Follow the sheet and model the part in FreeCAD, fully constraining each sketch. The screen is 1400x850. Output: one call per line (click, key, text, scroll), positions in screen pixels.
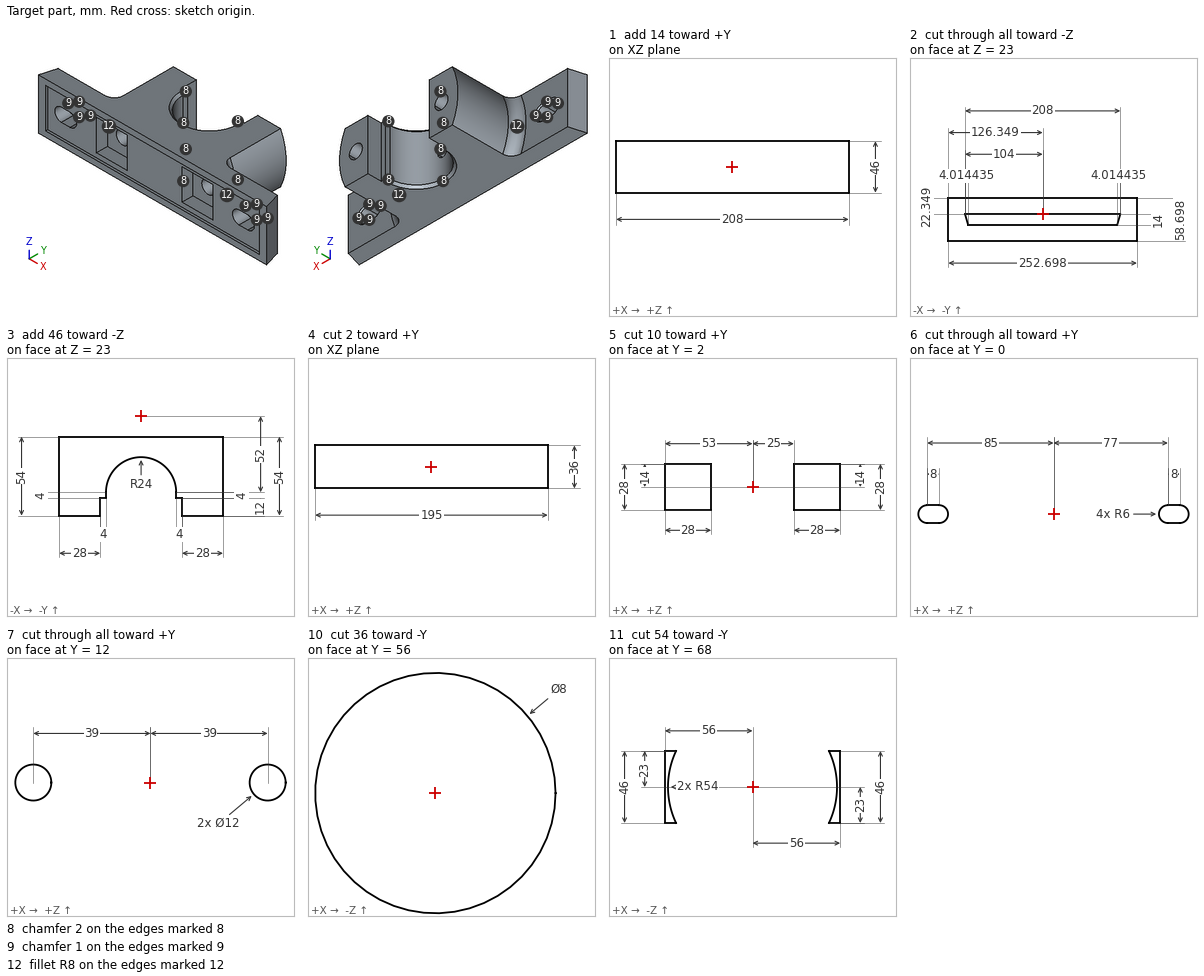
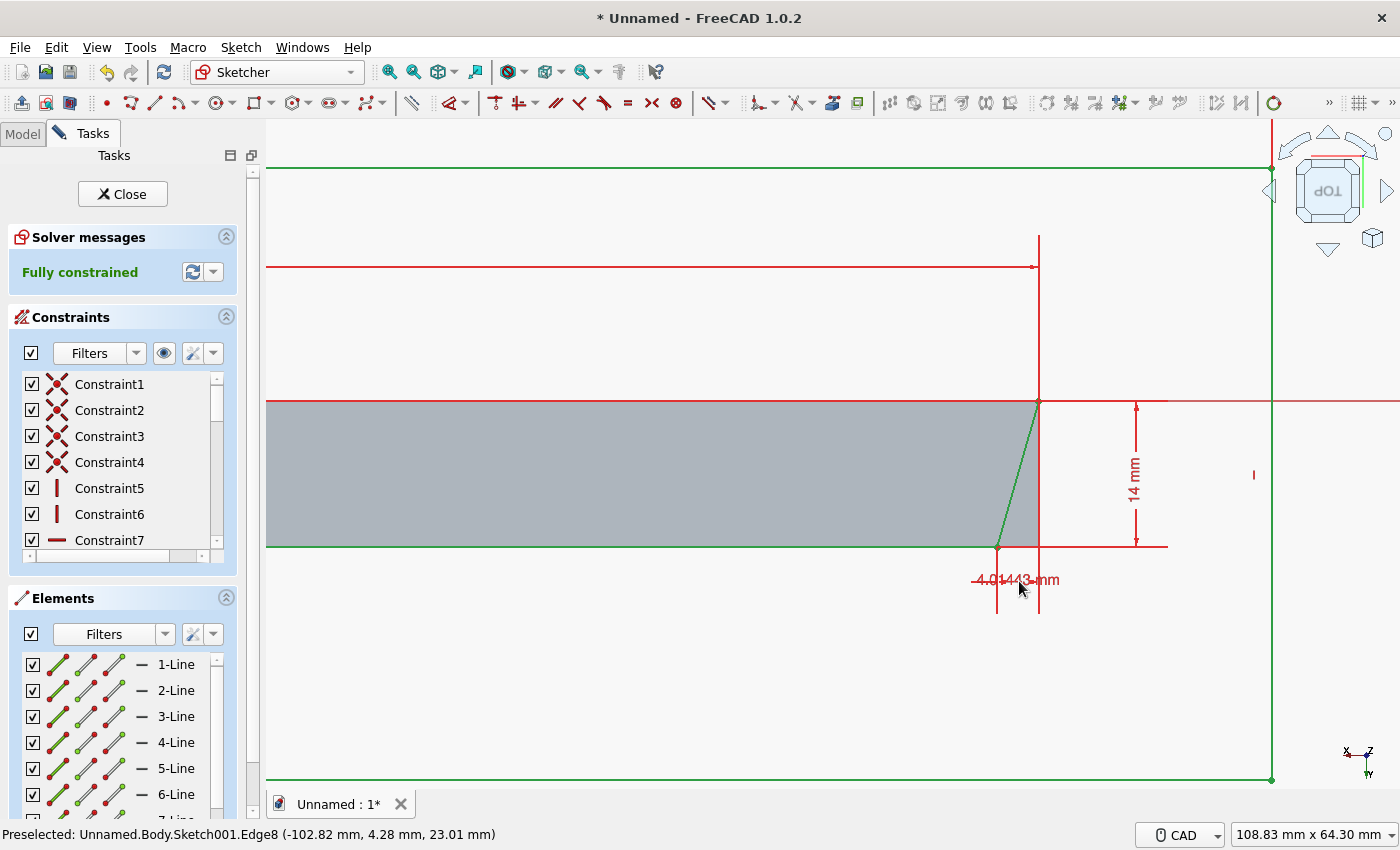
click(123, 194)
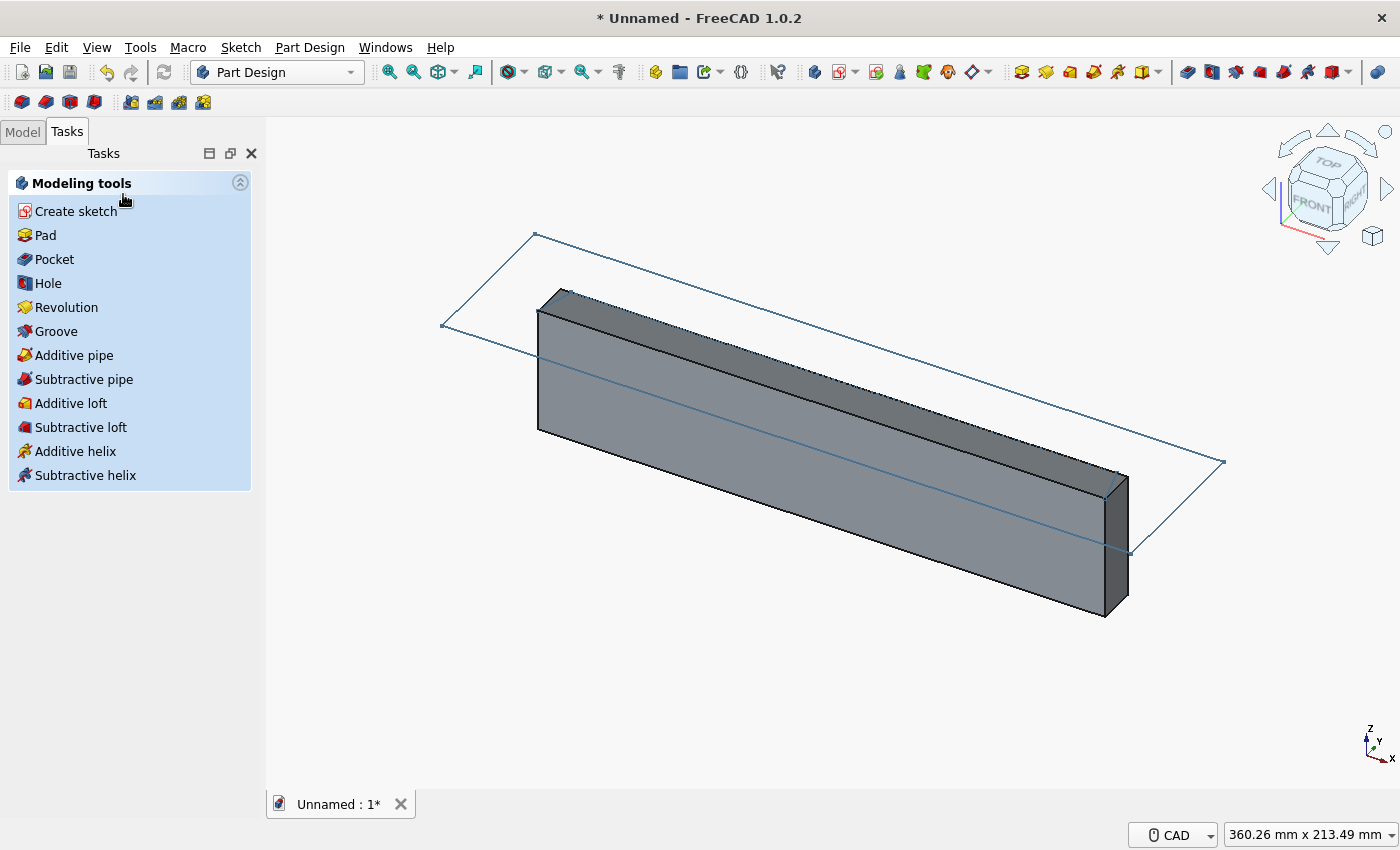
click(1188, 72)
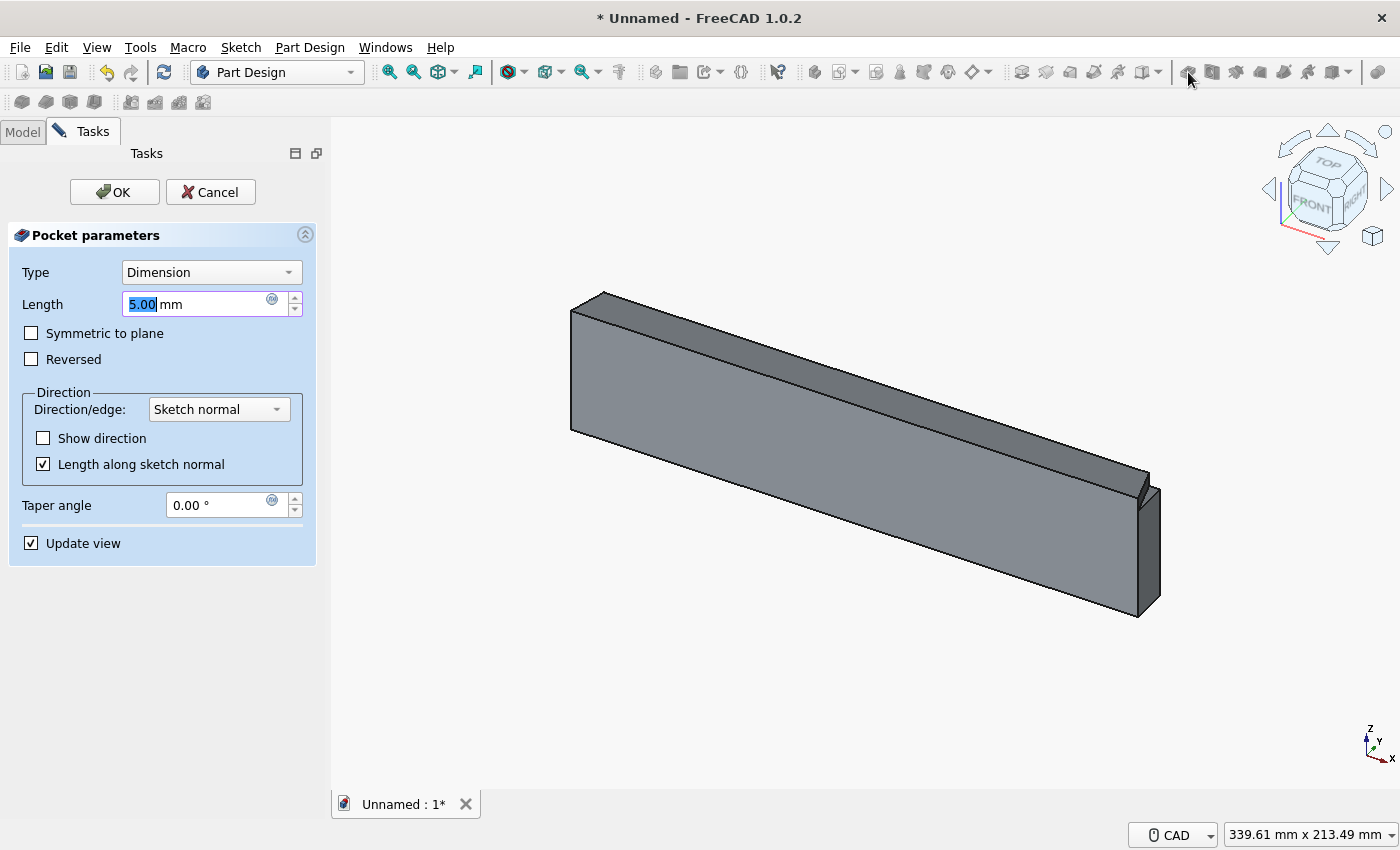
click(212, 272)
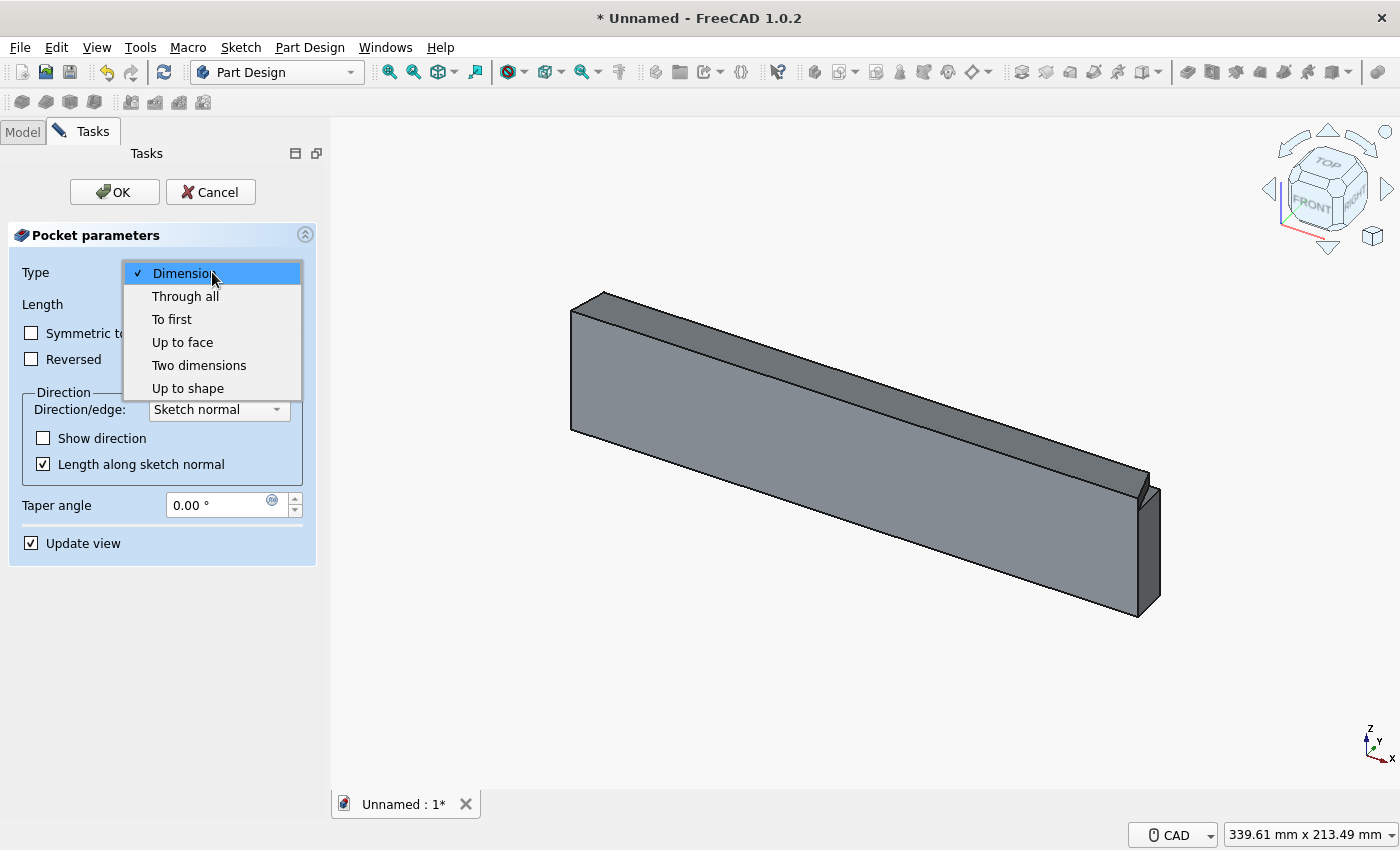
click(212, 296)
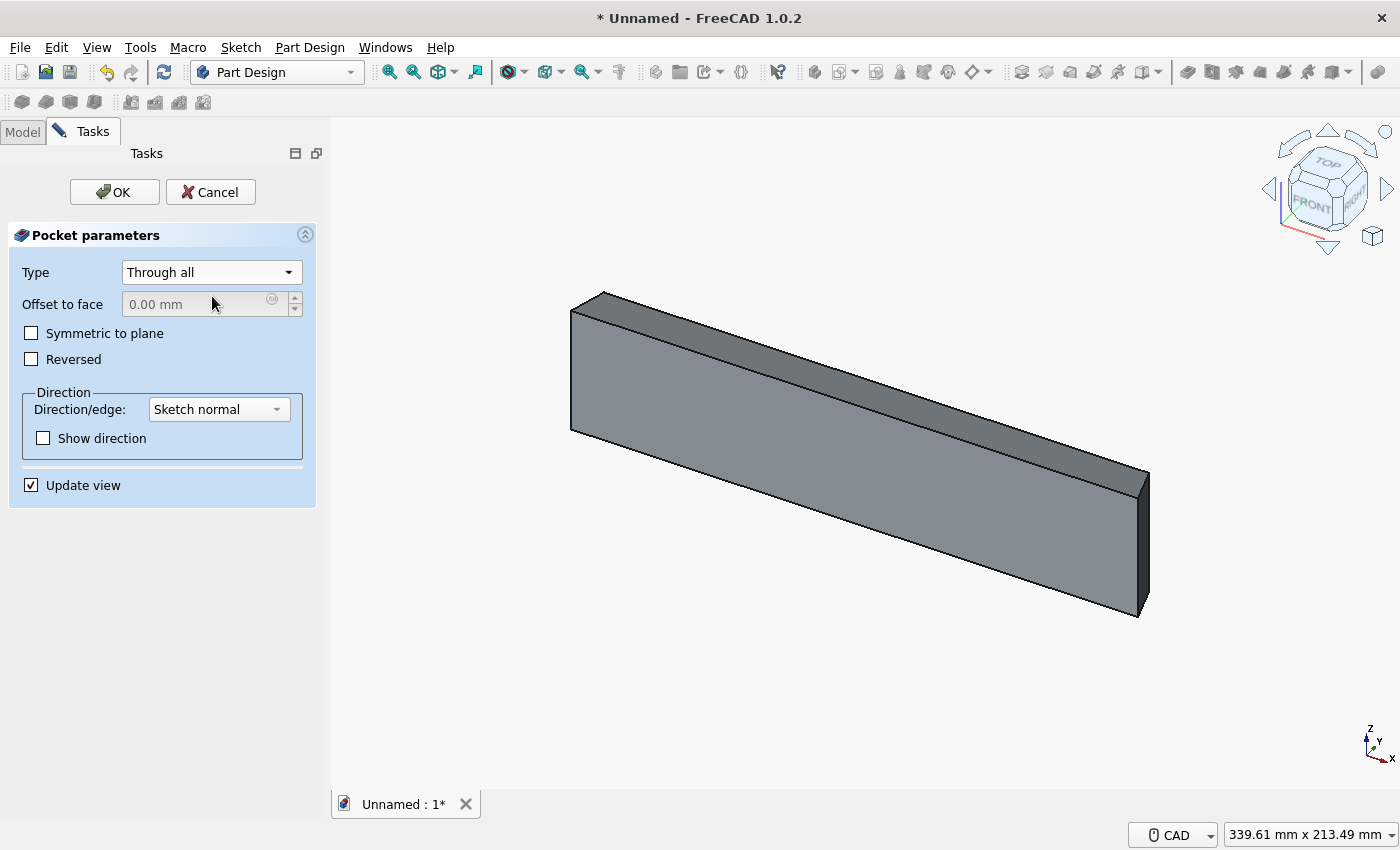
click(115, 192)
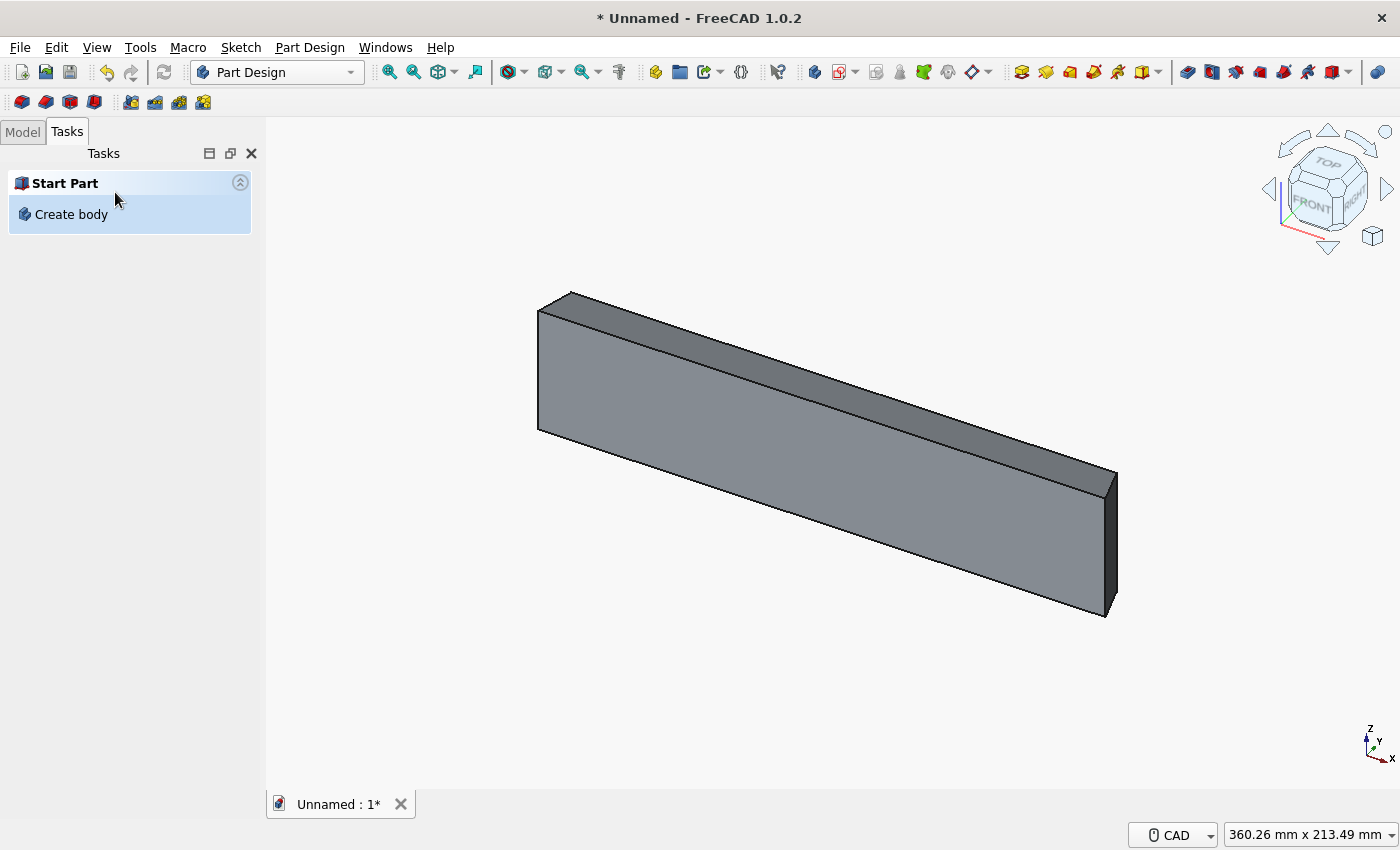
click(1076, 473)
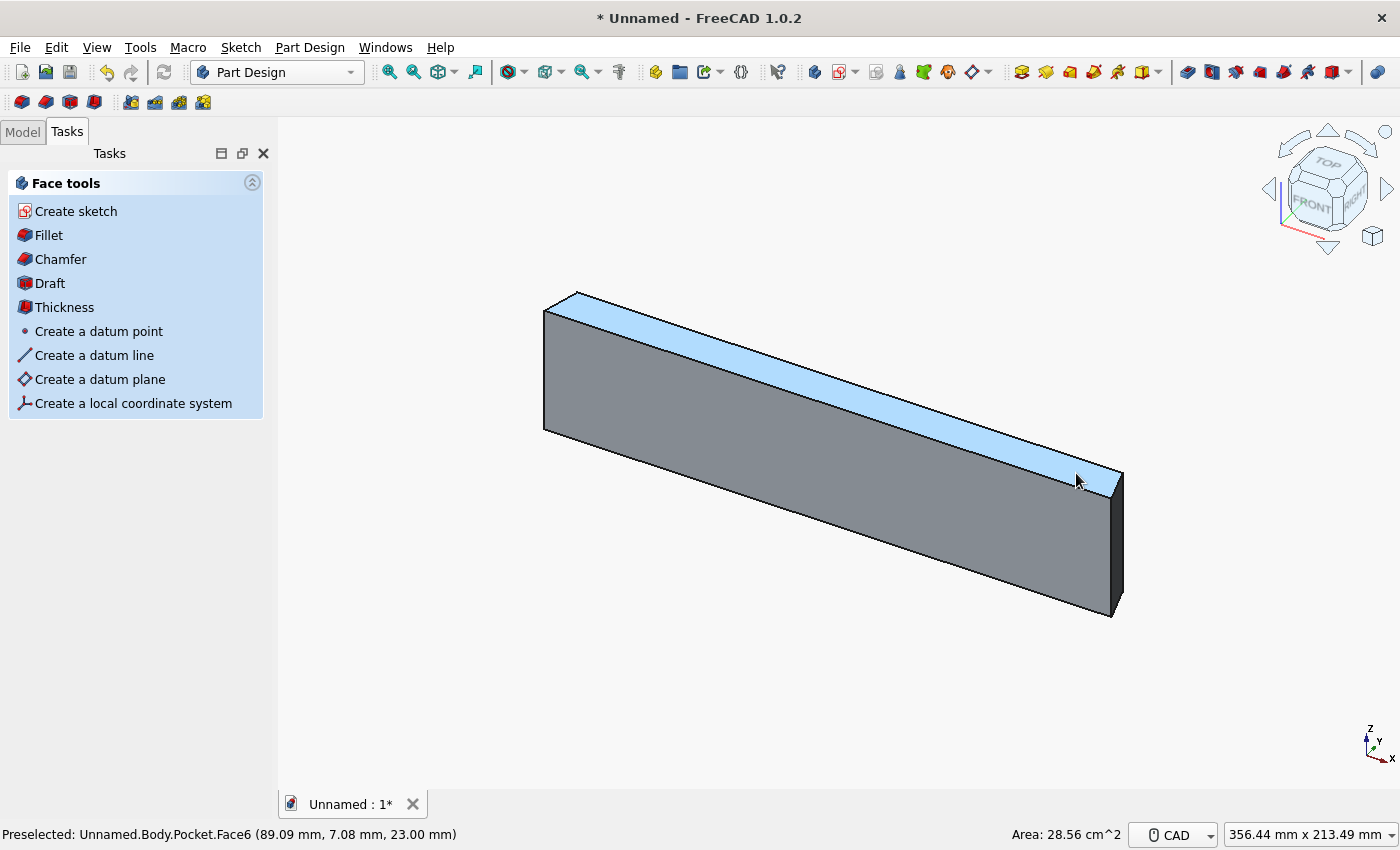
click(840, 72)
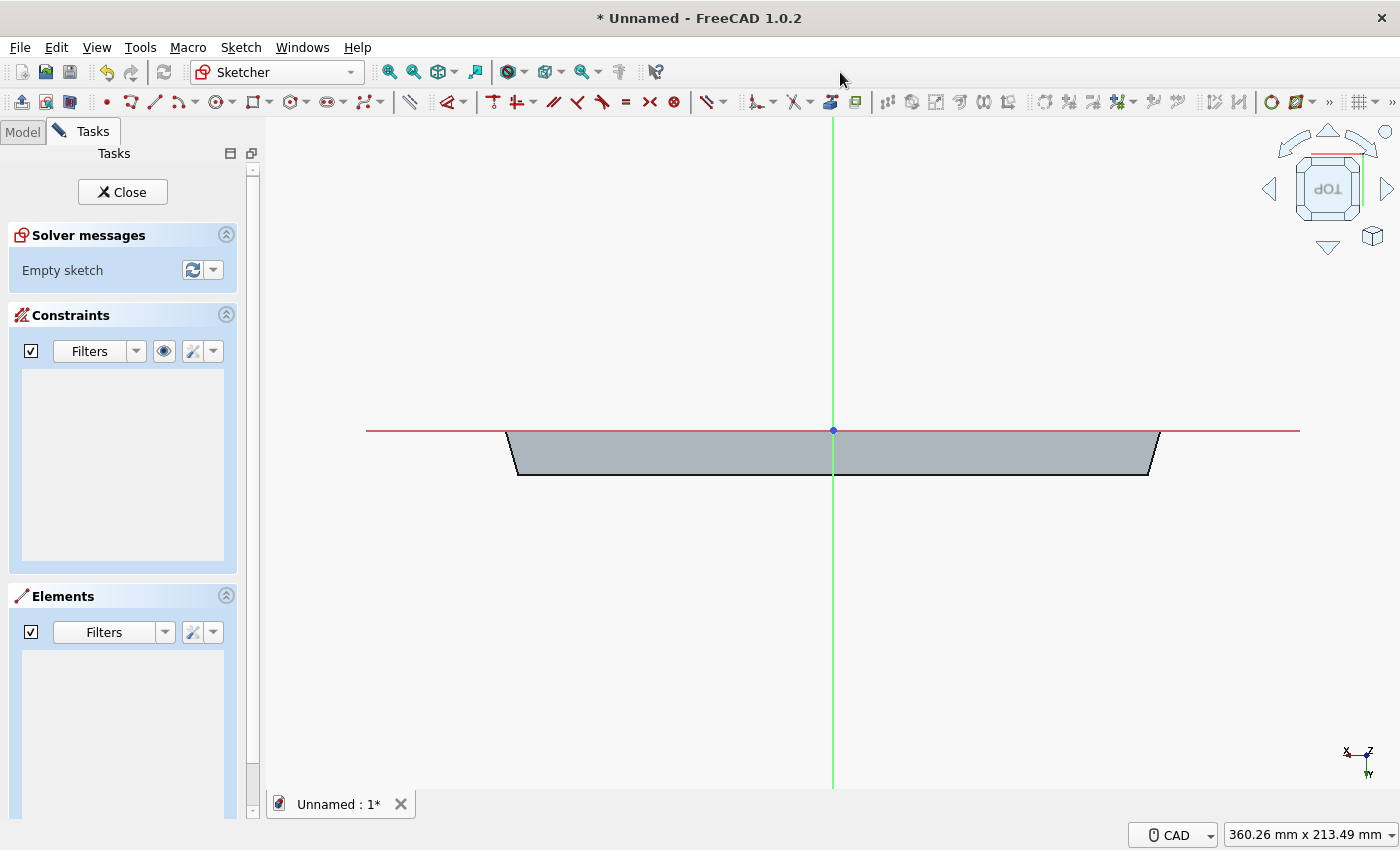
scroll(916, 641, up, 3)